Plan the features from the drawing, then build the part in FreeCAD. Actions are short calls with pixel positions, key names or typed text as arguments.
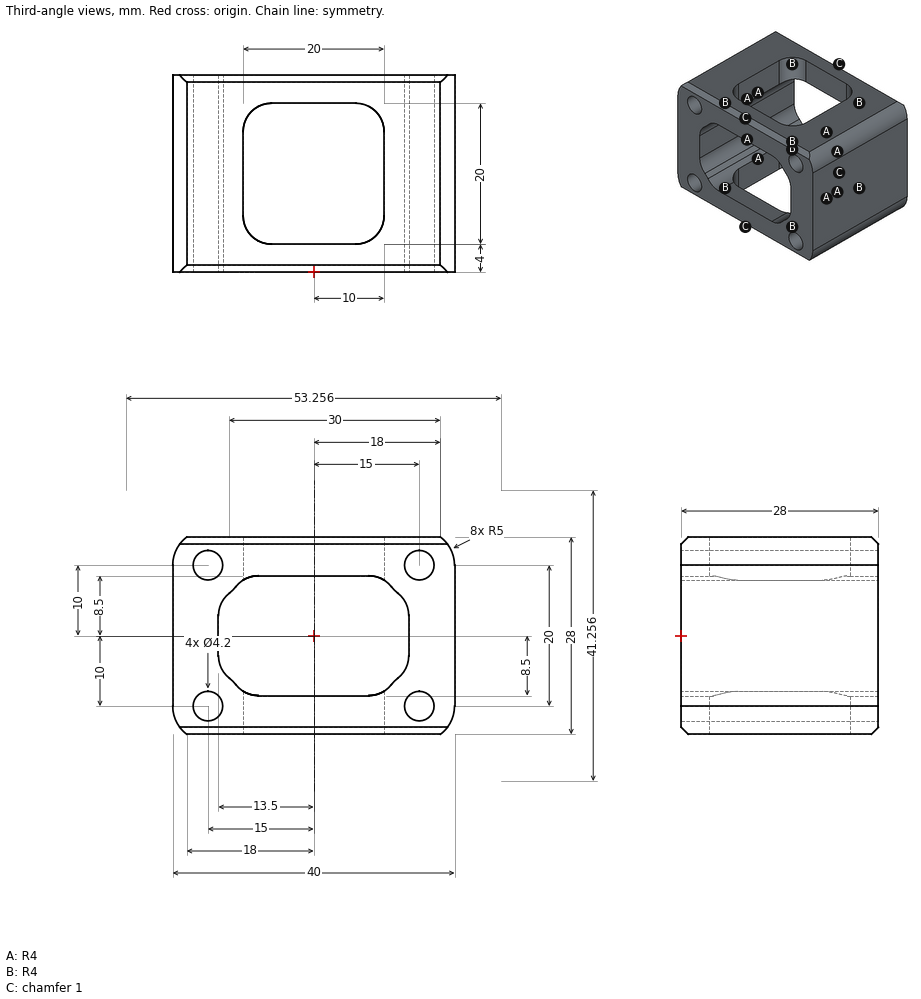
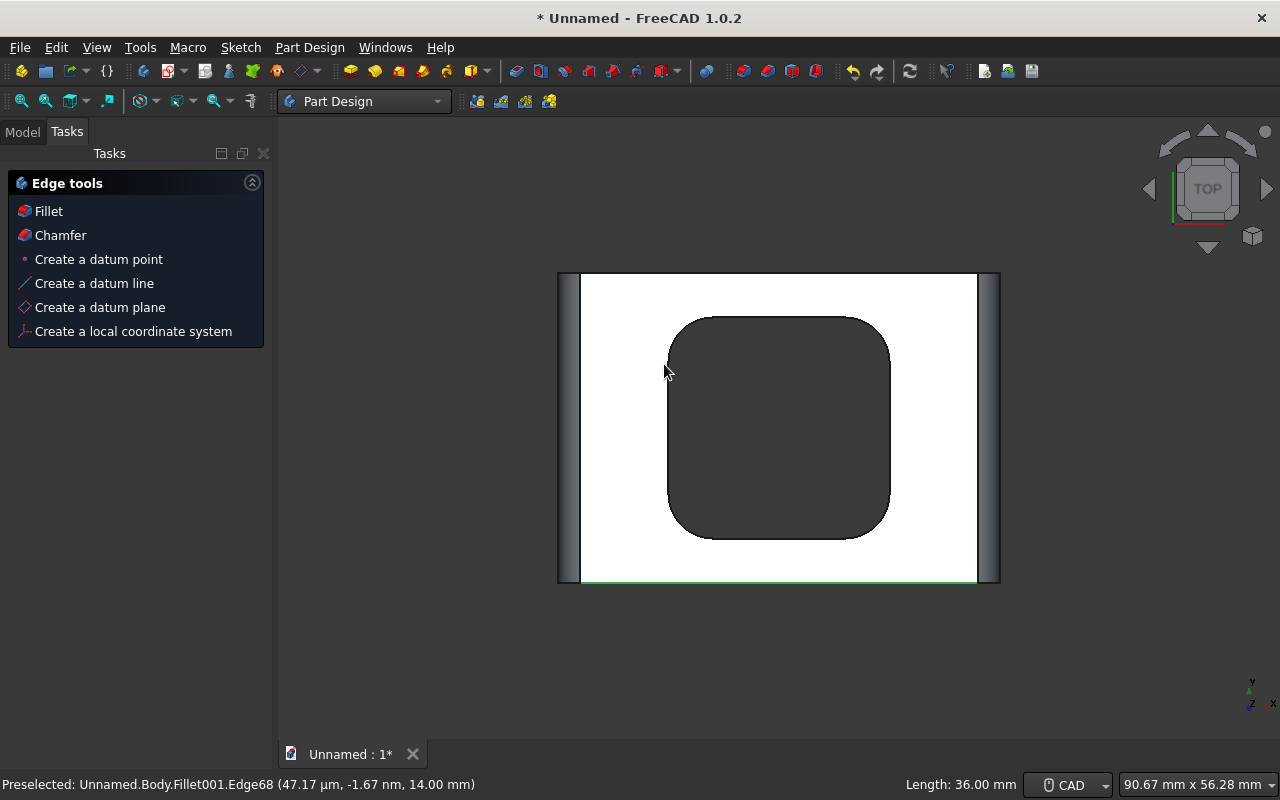
click(779, 272, ctrl)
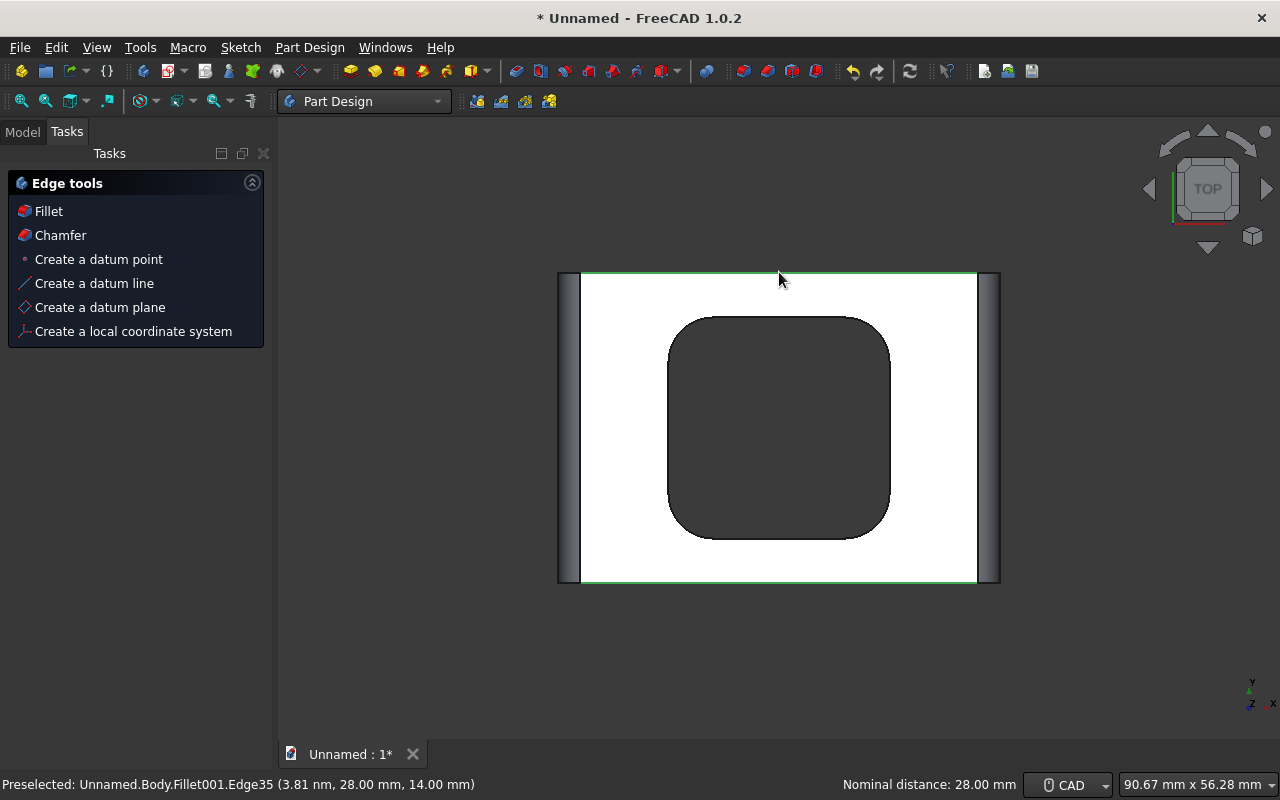
key(0)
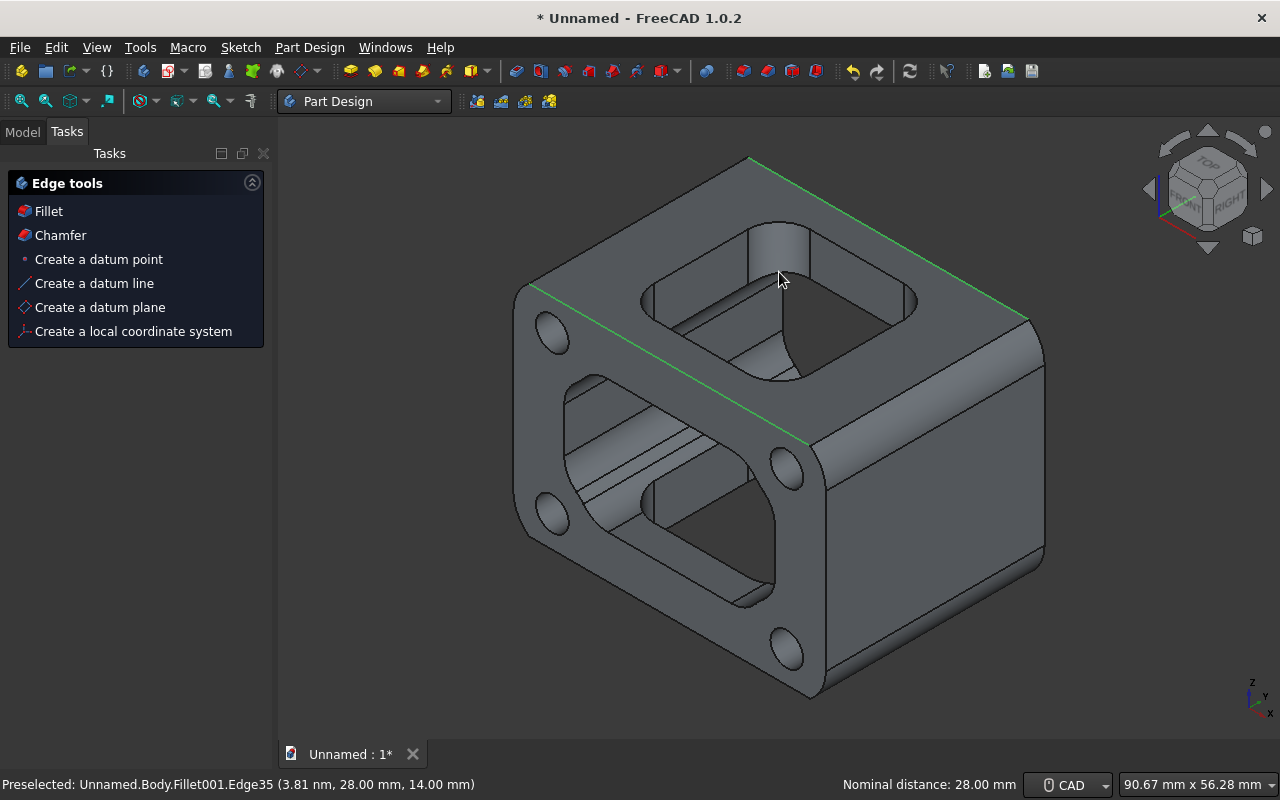
key(1)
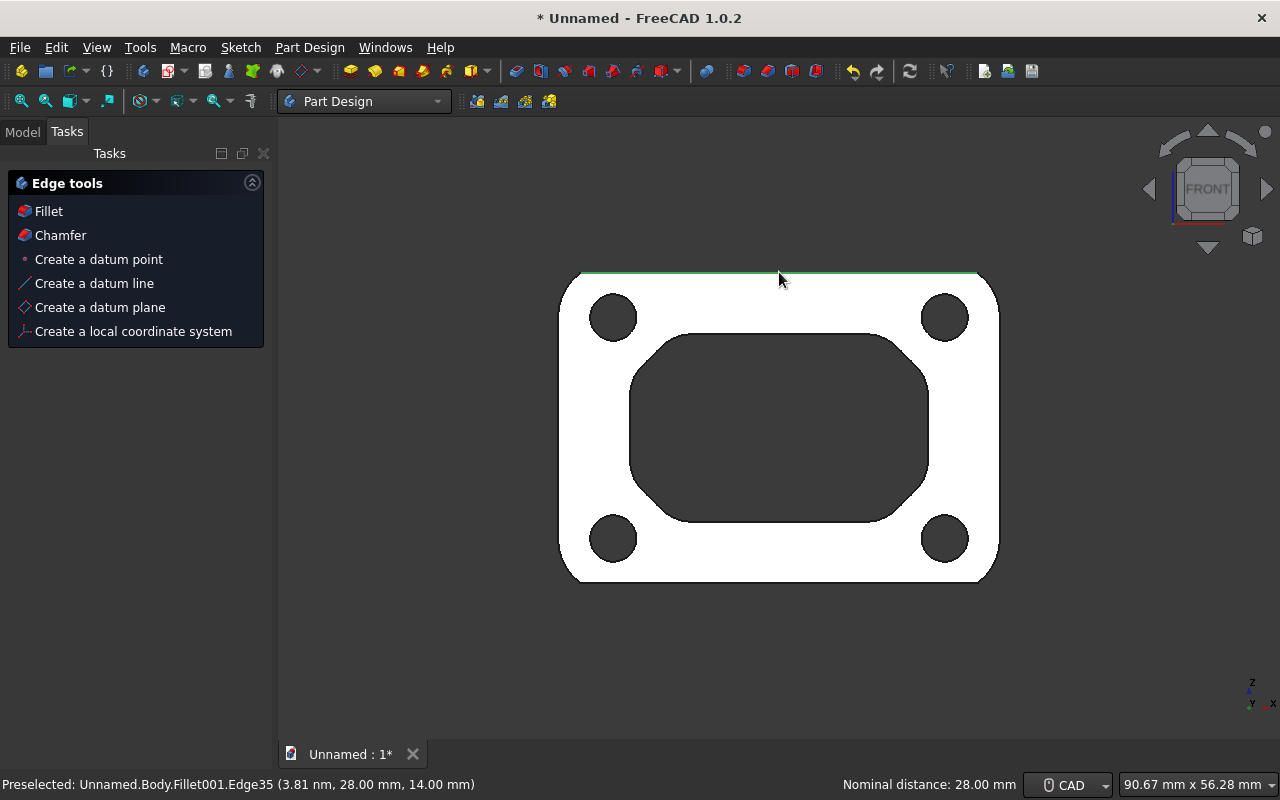
key(3)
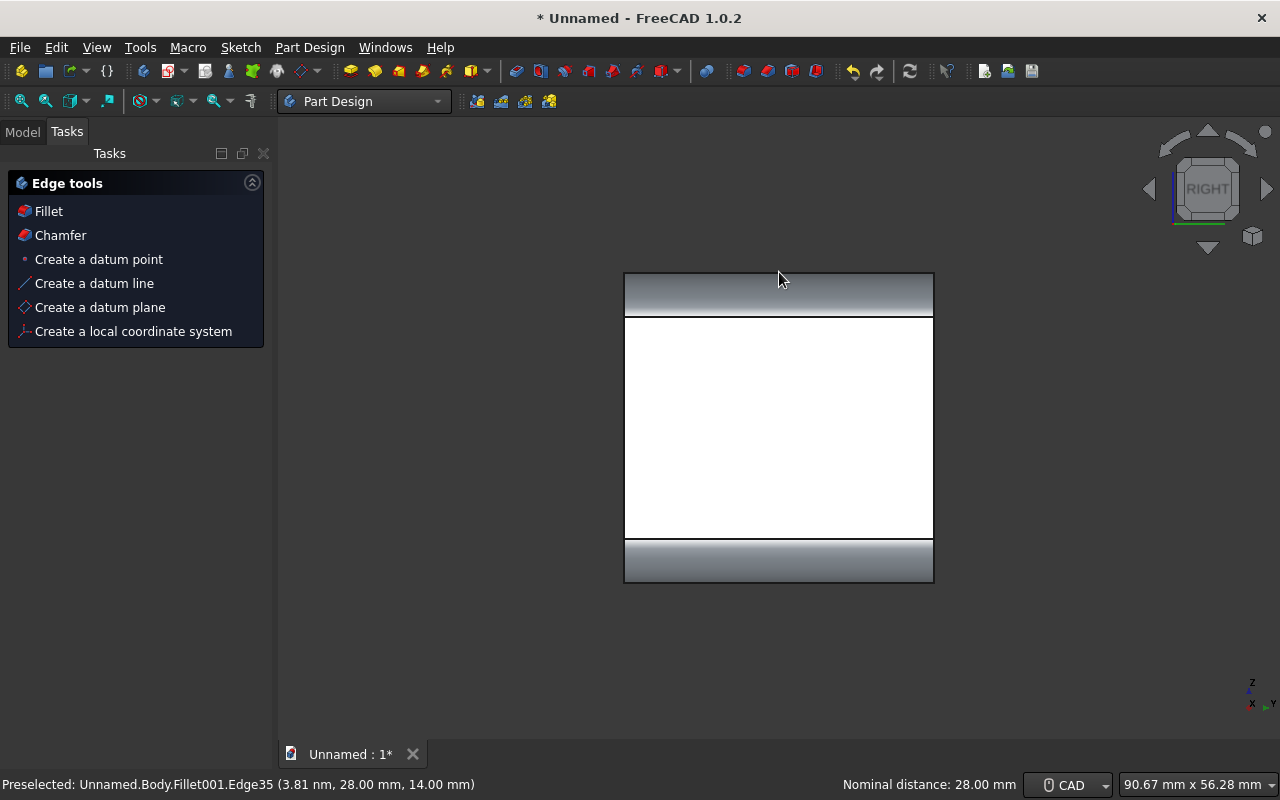
key(5)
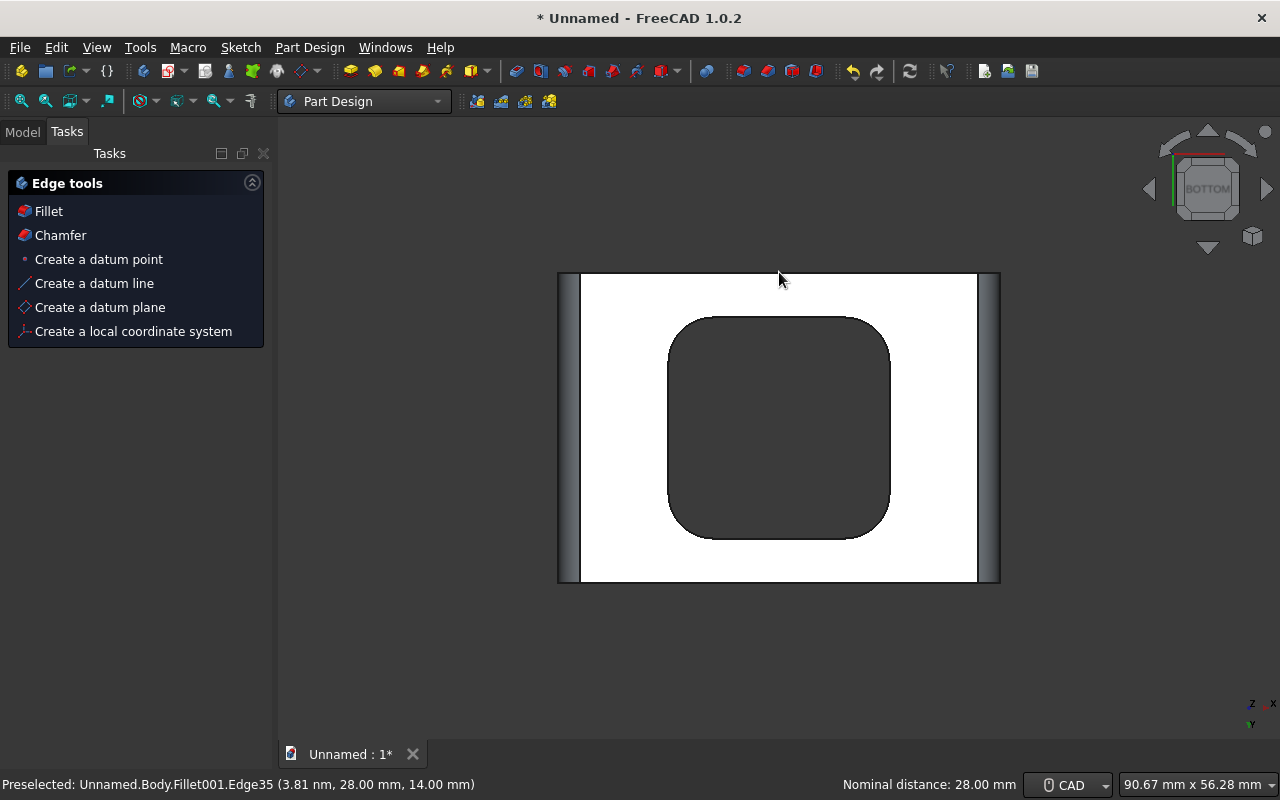
click(779, 272, ctrl)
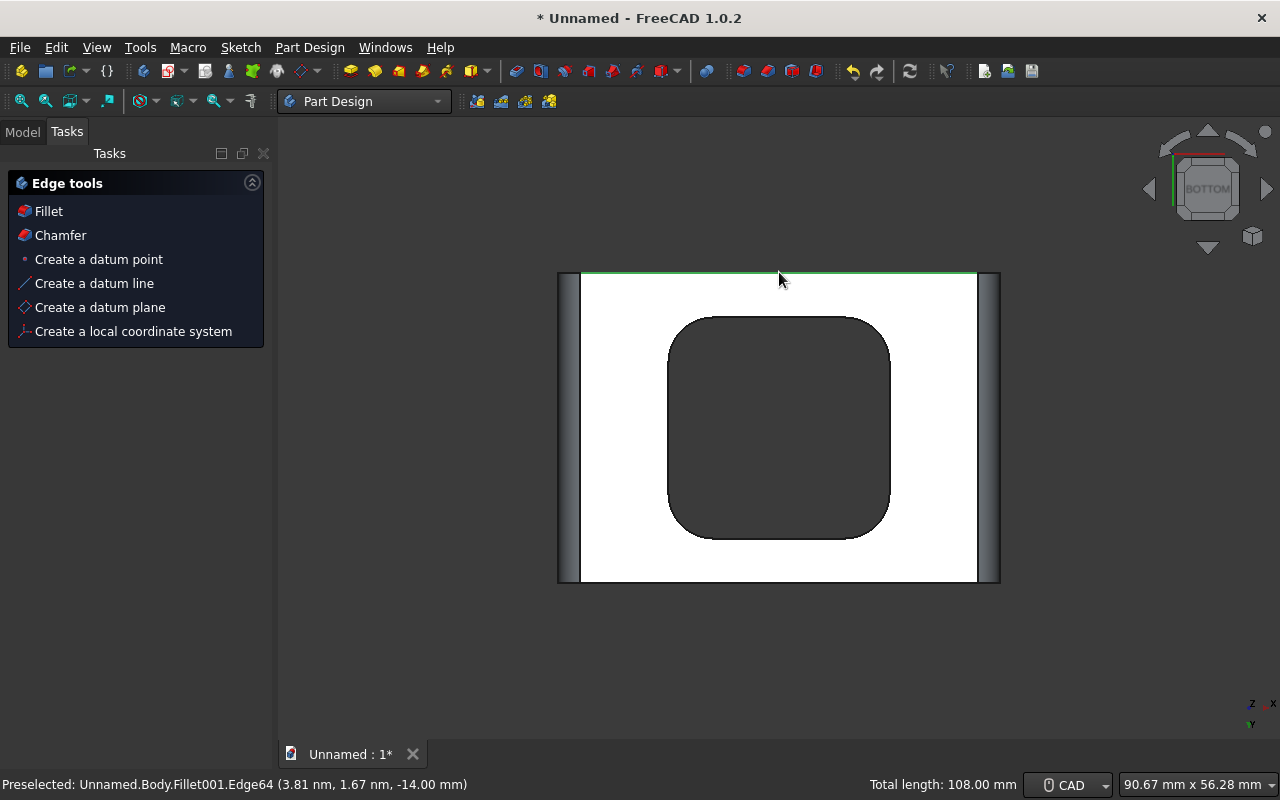
key(4)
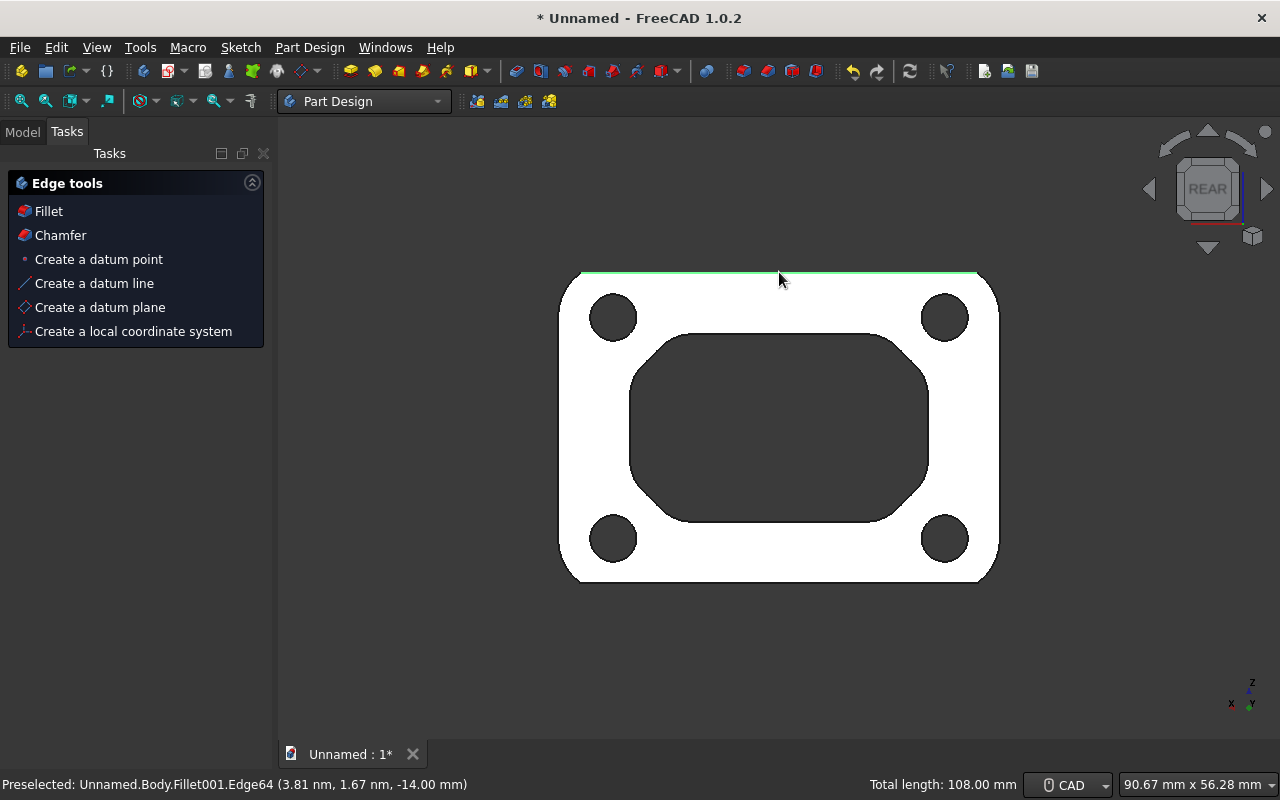
click(779, 582, ctrl)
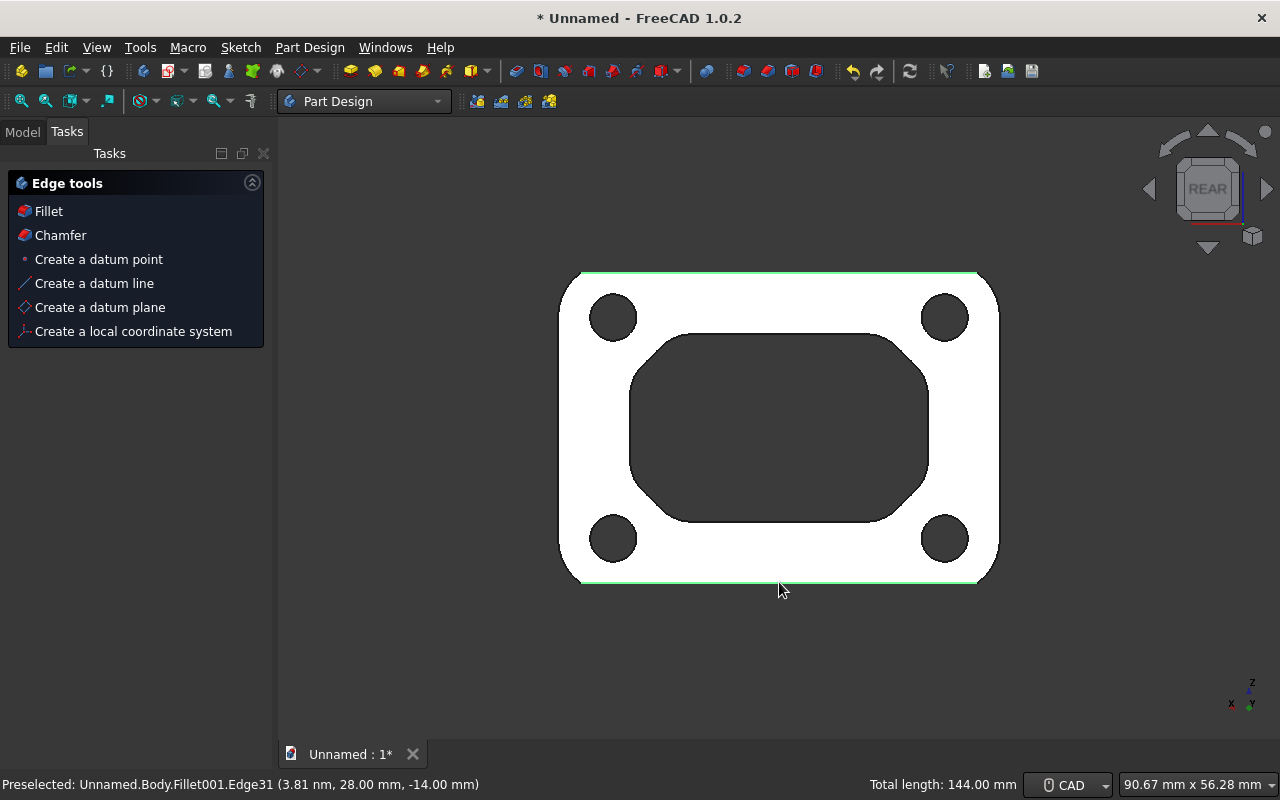
click(768, 72)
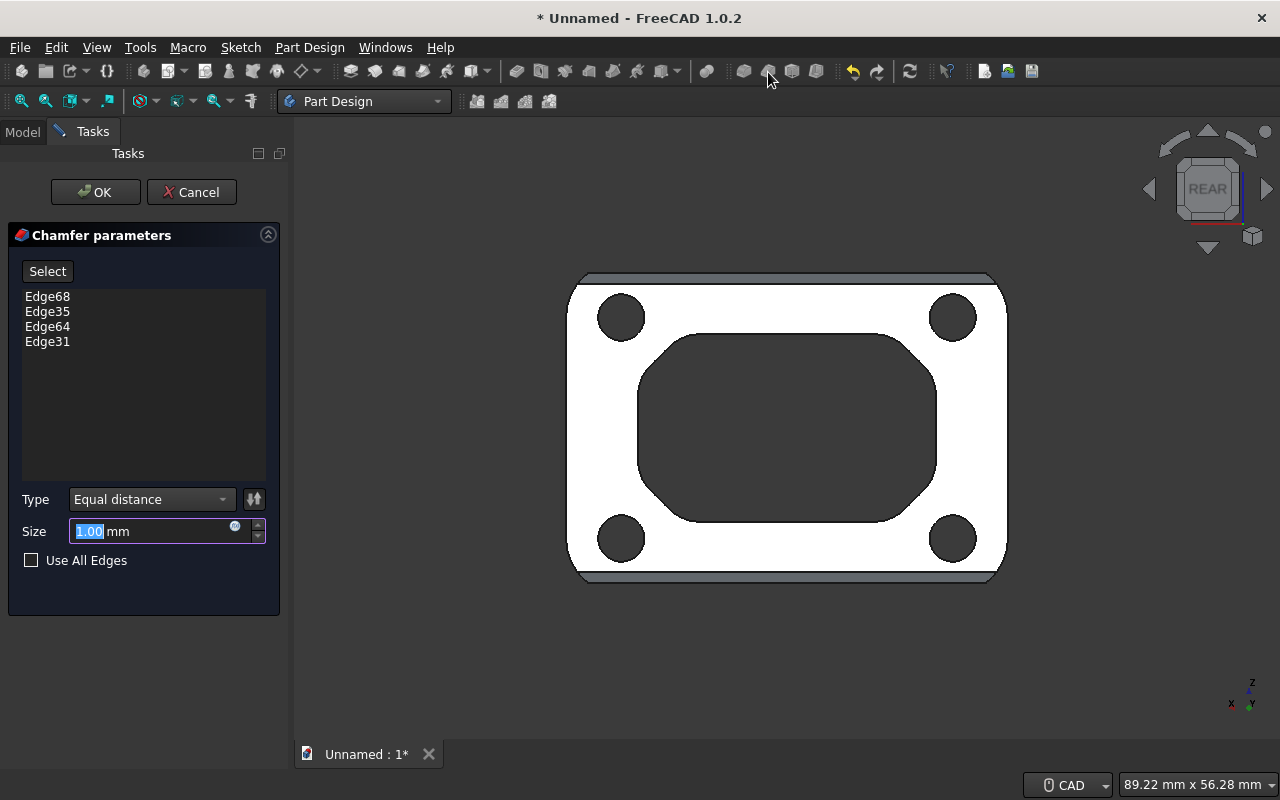
text(1)
key(Tab)